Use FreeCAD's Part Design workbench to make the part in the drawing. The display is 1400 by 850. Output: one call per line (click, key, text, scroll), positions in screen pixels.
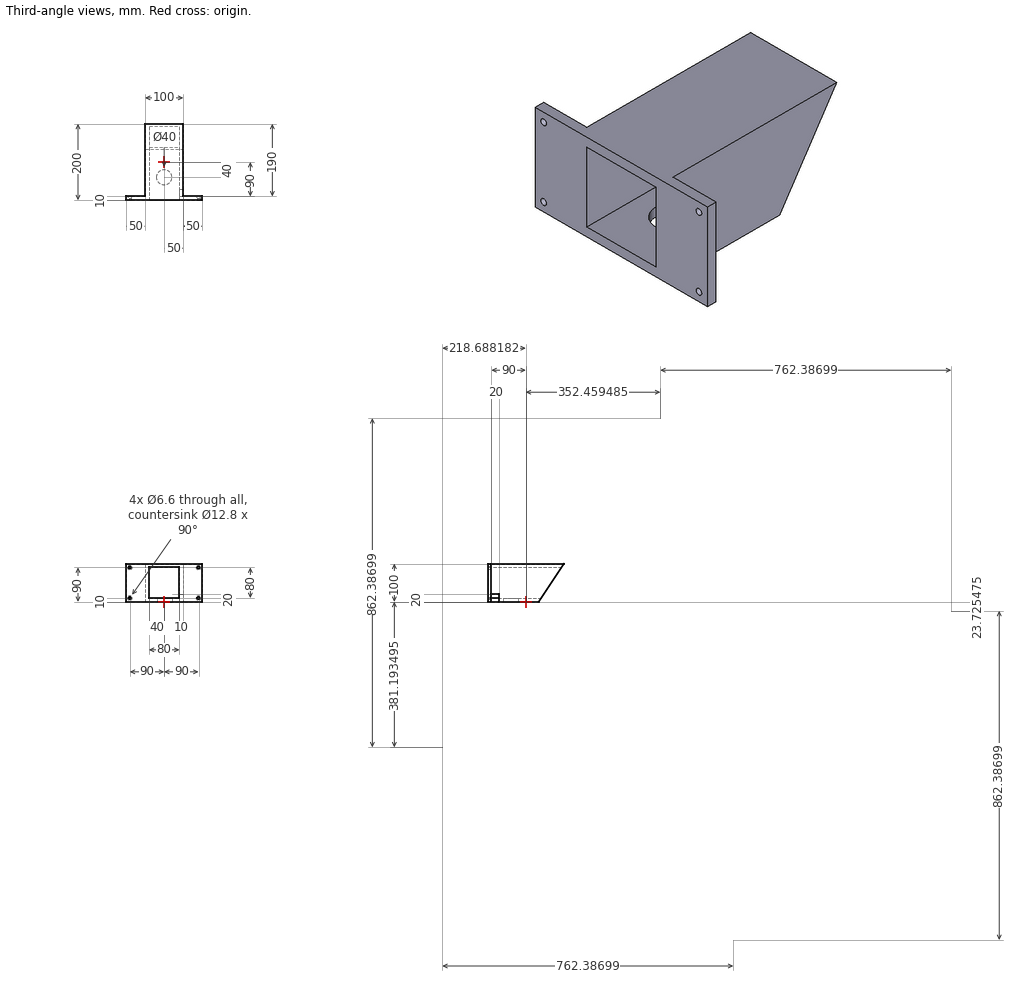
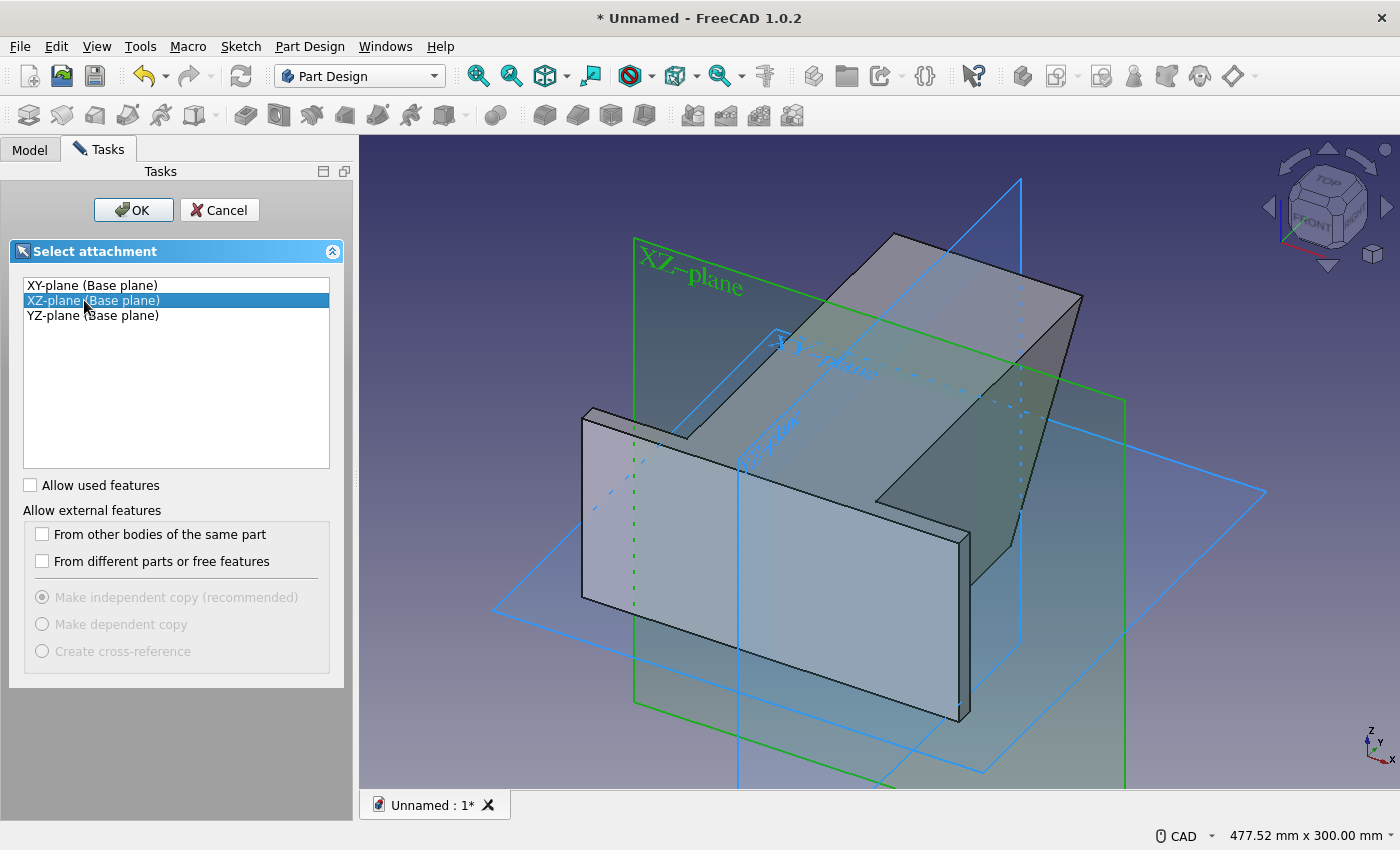
click(134, 210)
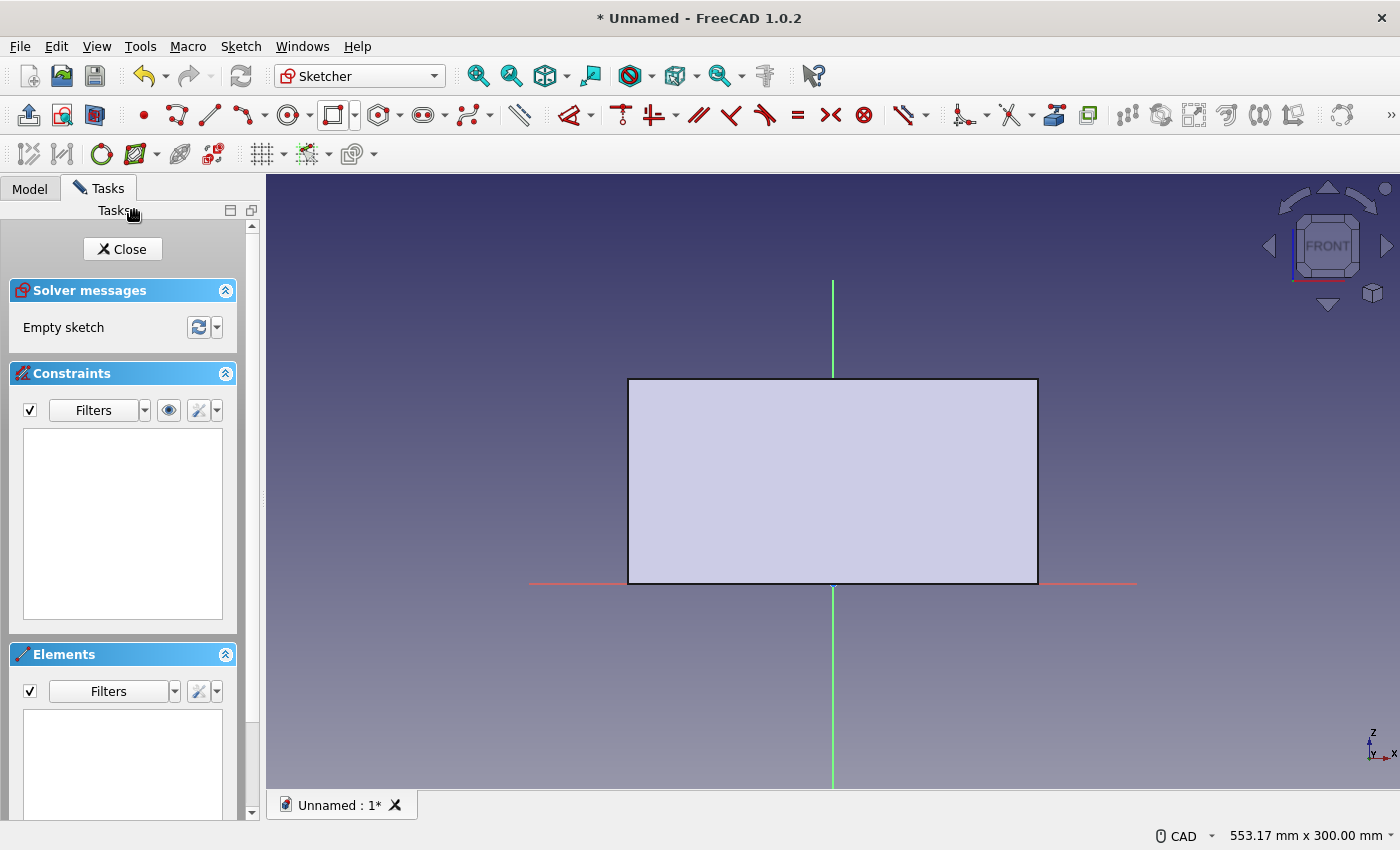
key(q)
key(s)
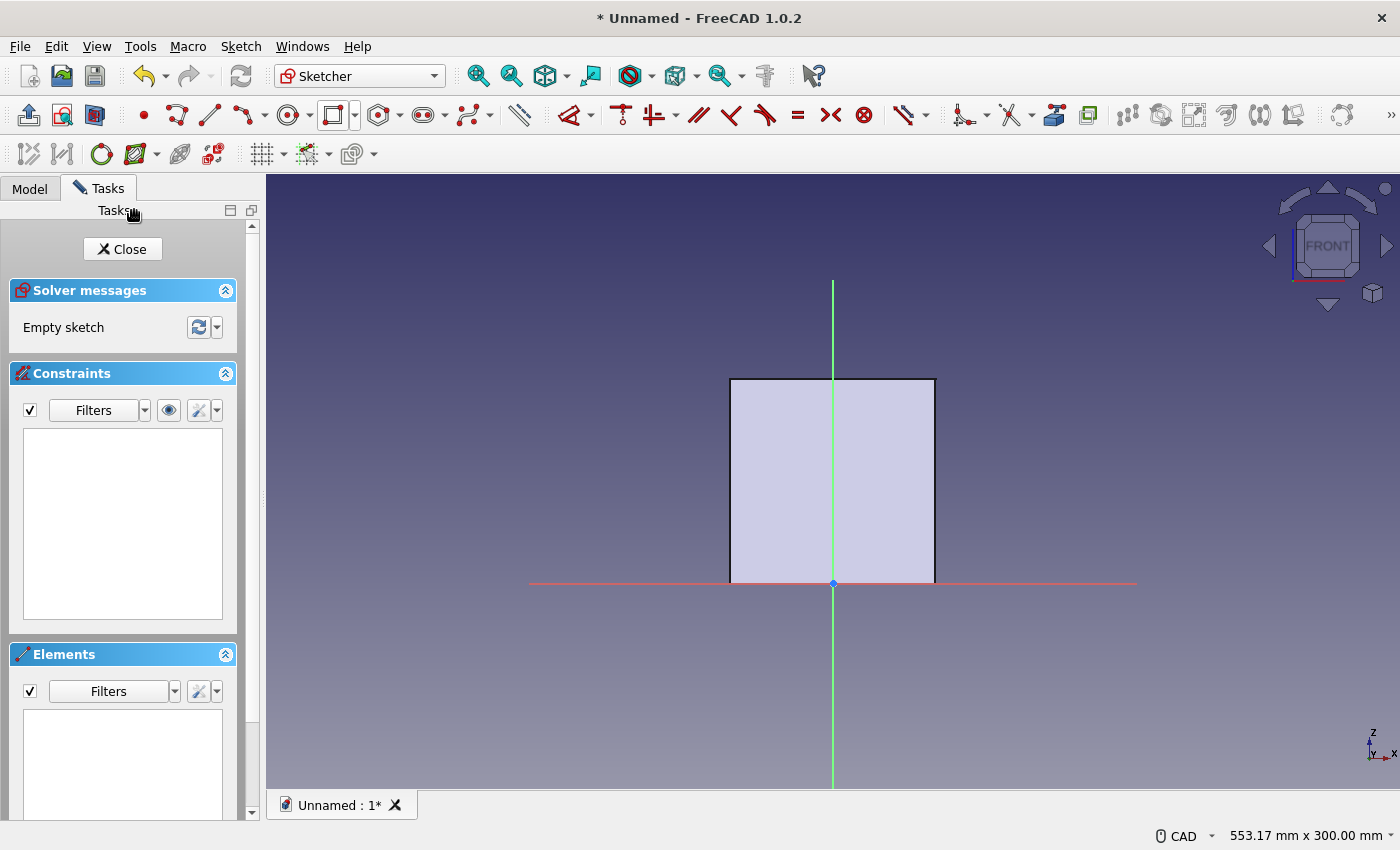
scroll(889, 500, up, 4)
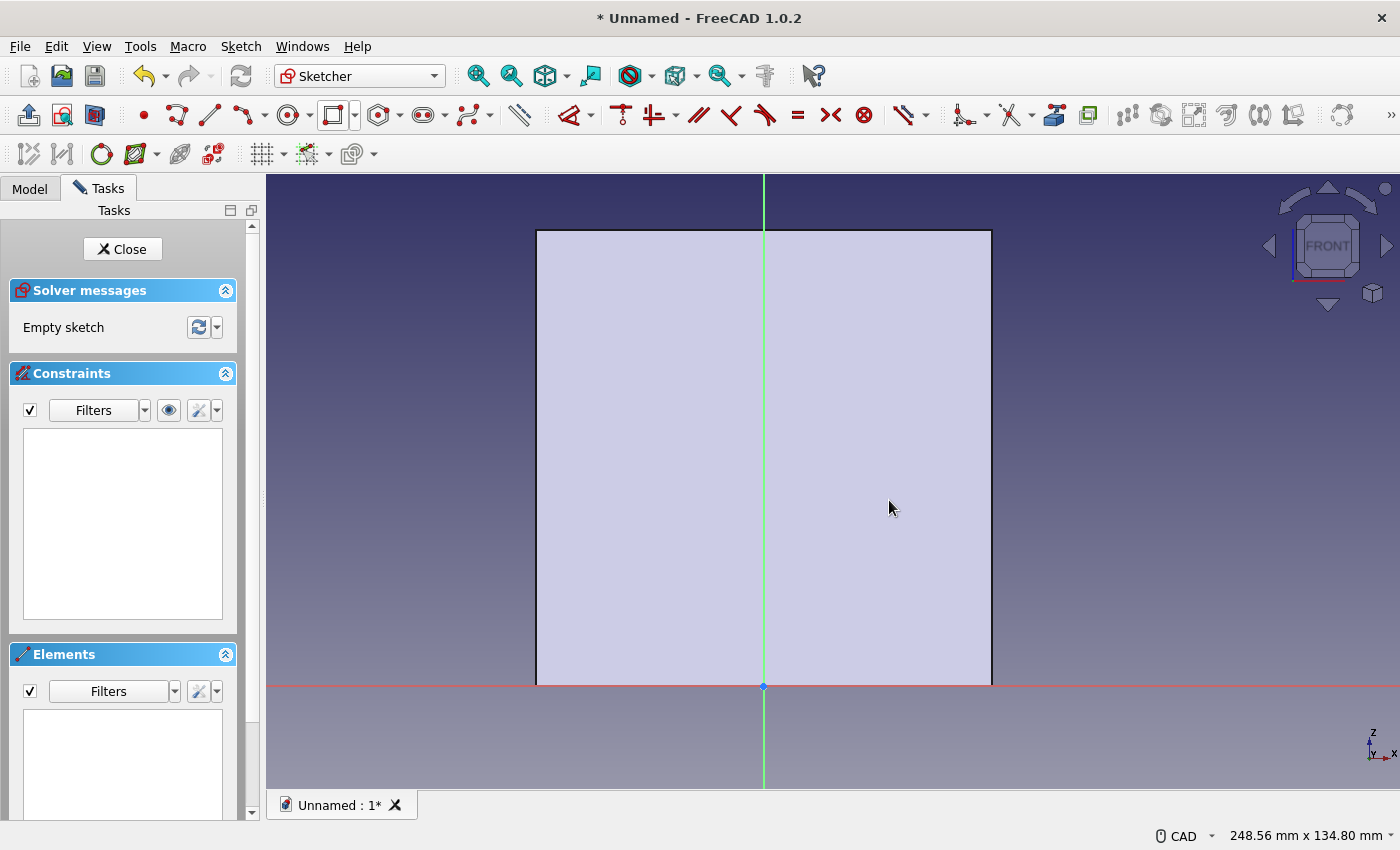
key(g)
key(r)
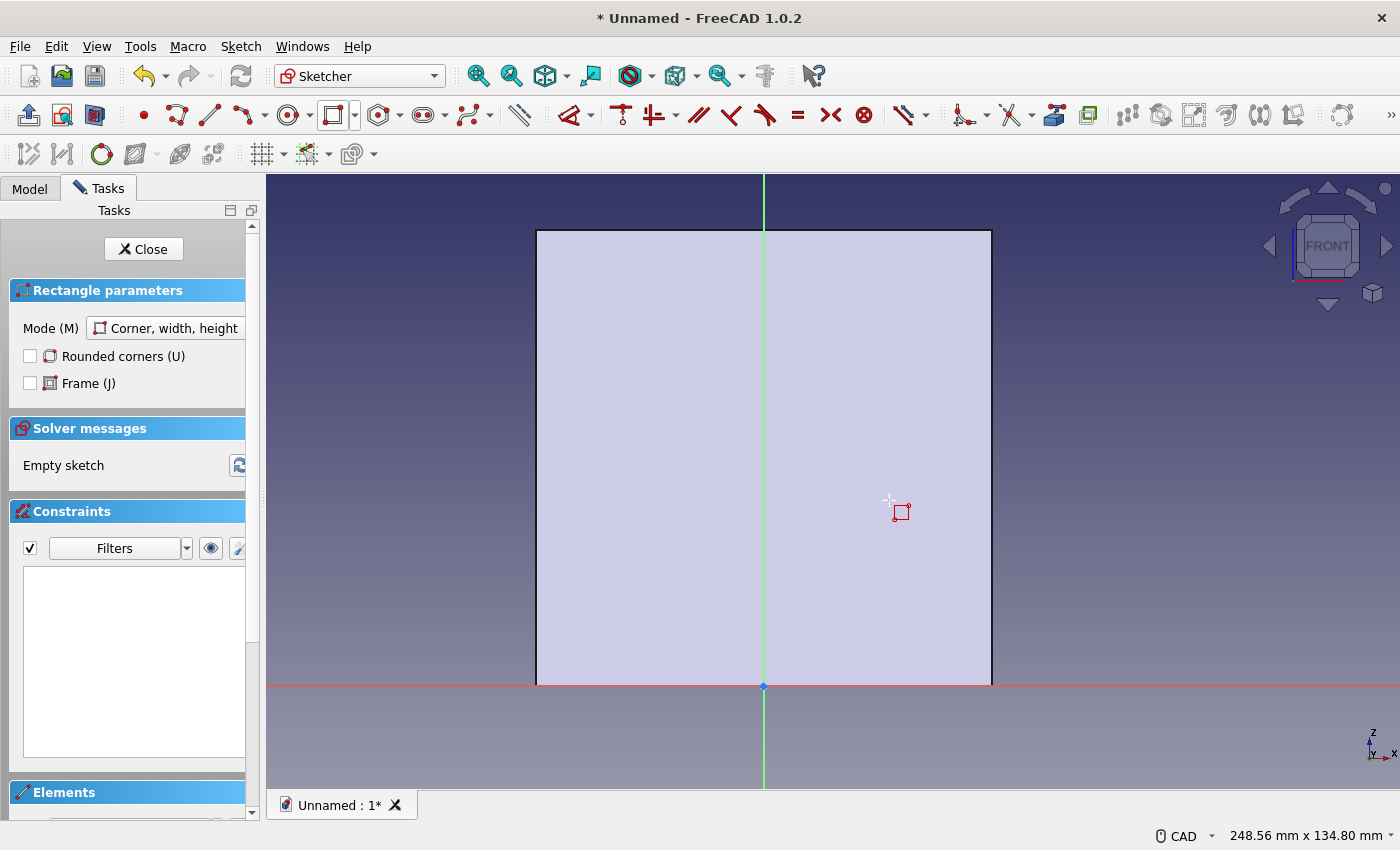
click(581, 276)
move(946, 641)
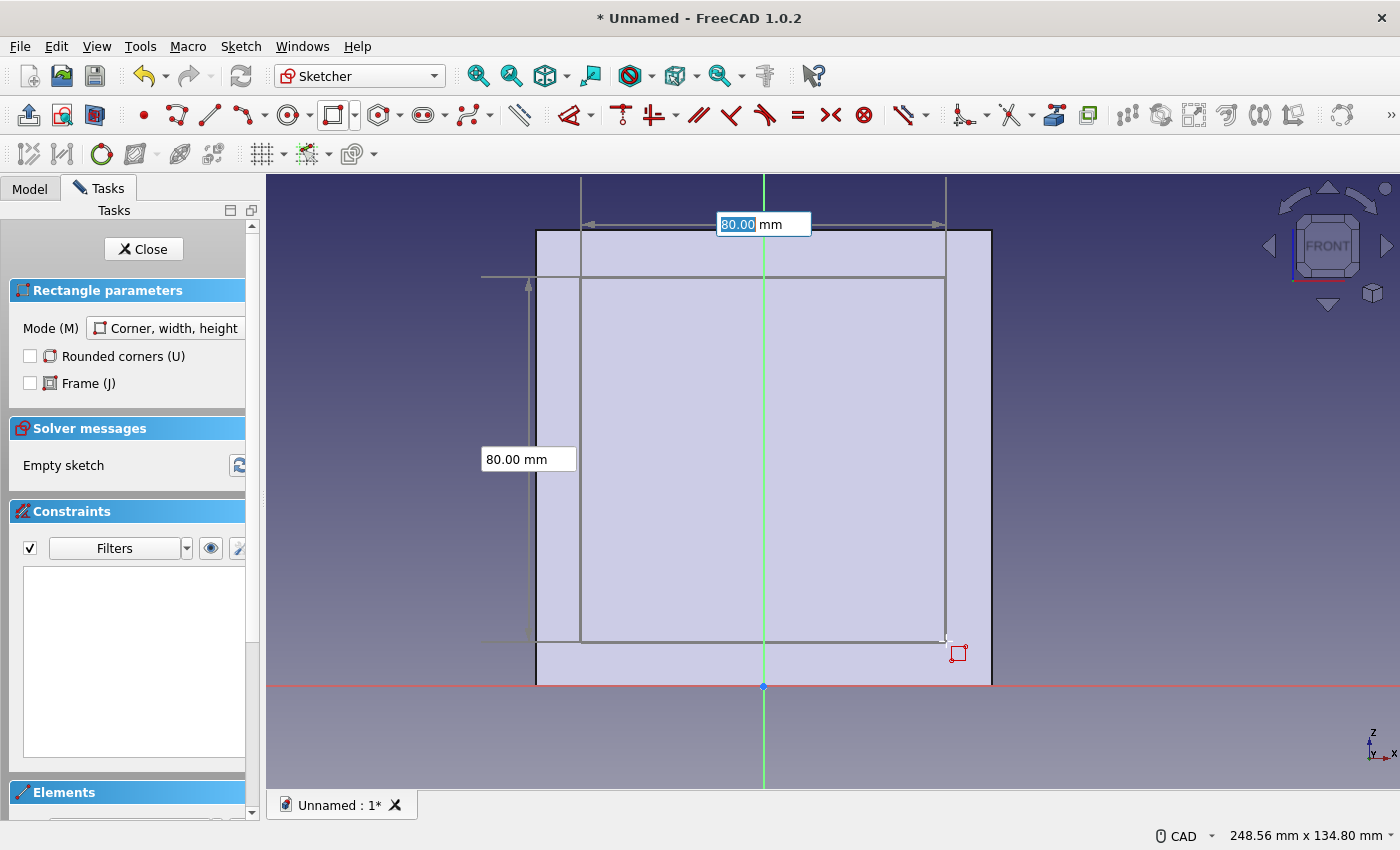
text(80)
key(Tab)
text(80)
key(Return)
key(Escape)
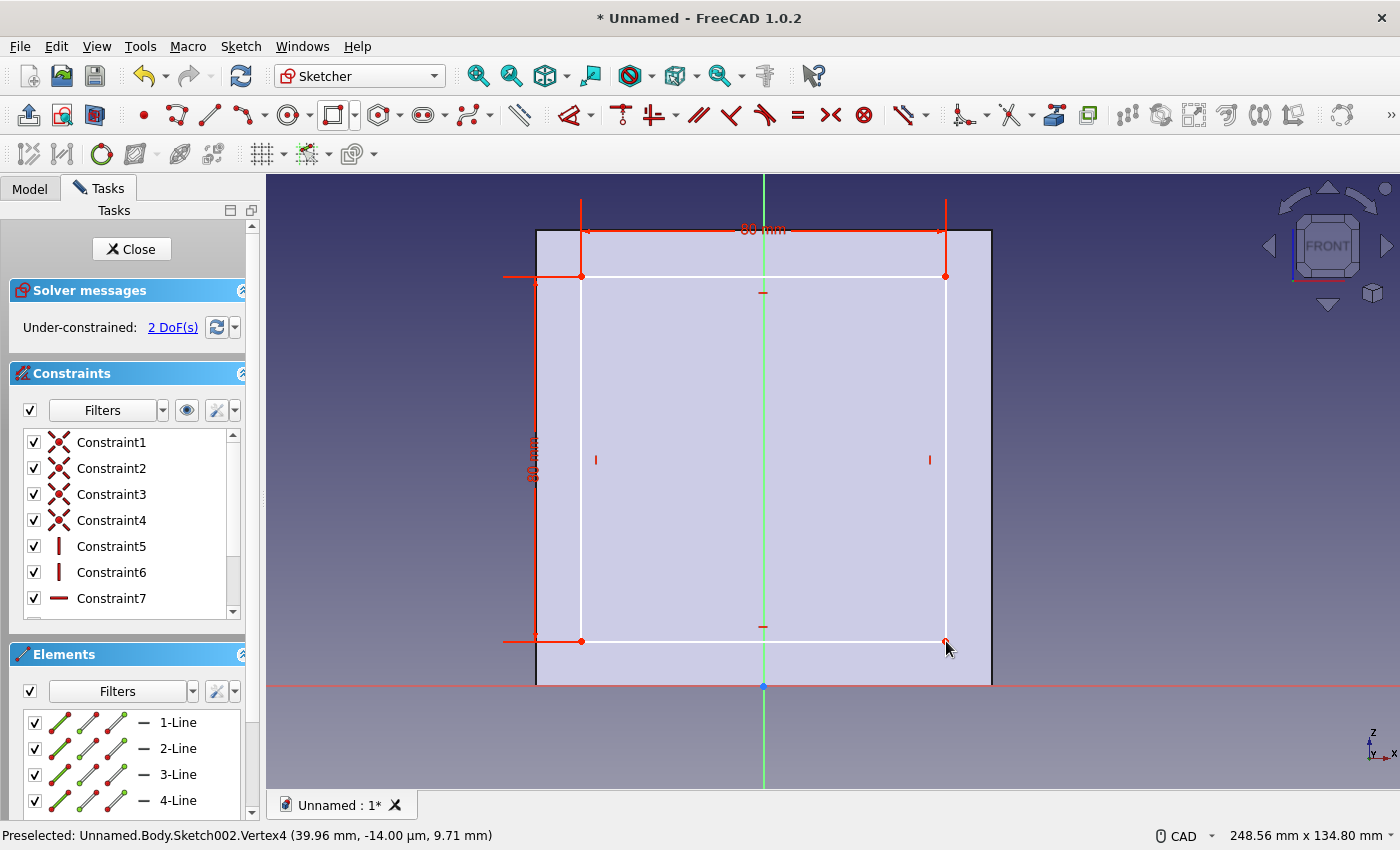
key(d)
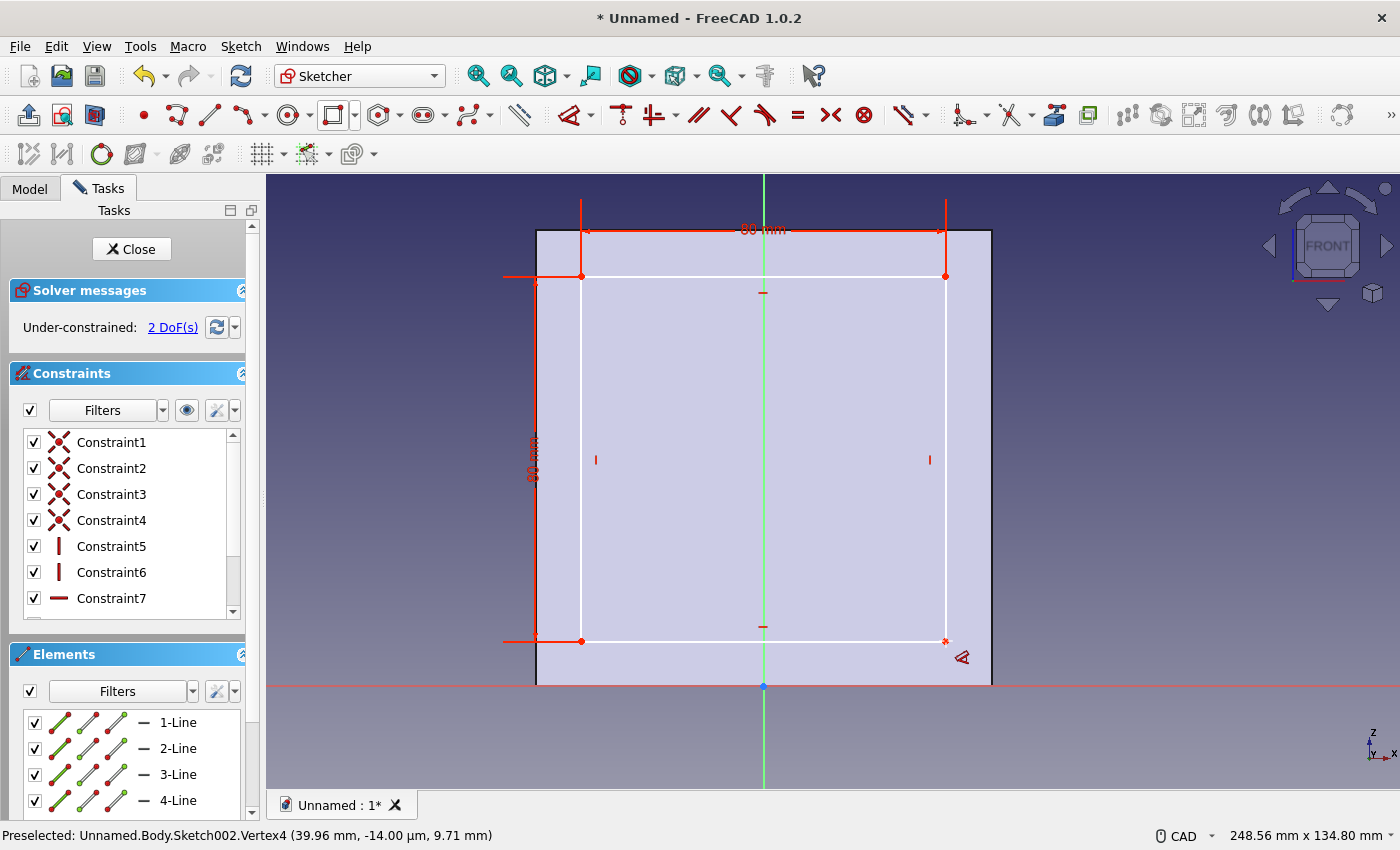
click(581, 277)
click(672, 720)